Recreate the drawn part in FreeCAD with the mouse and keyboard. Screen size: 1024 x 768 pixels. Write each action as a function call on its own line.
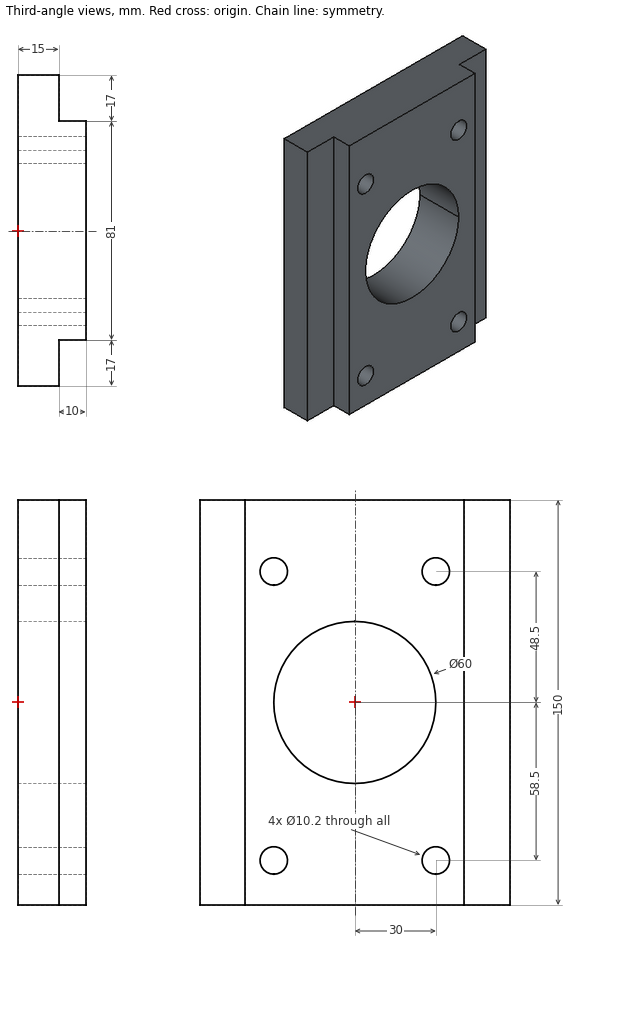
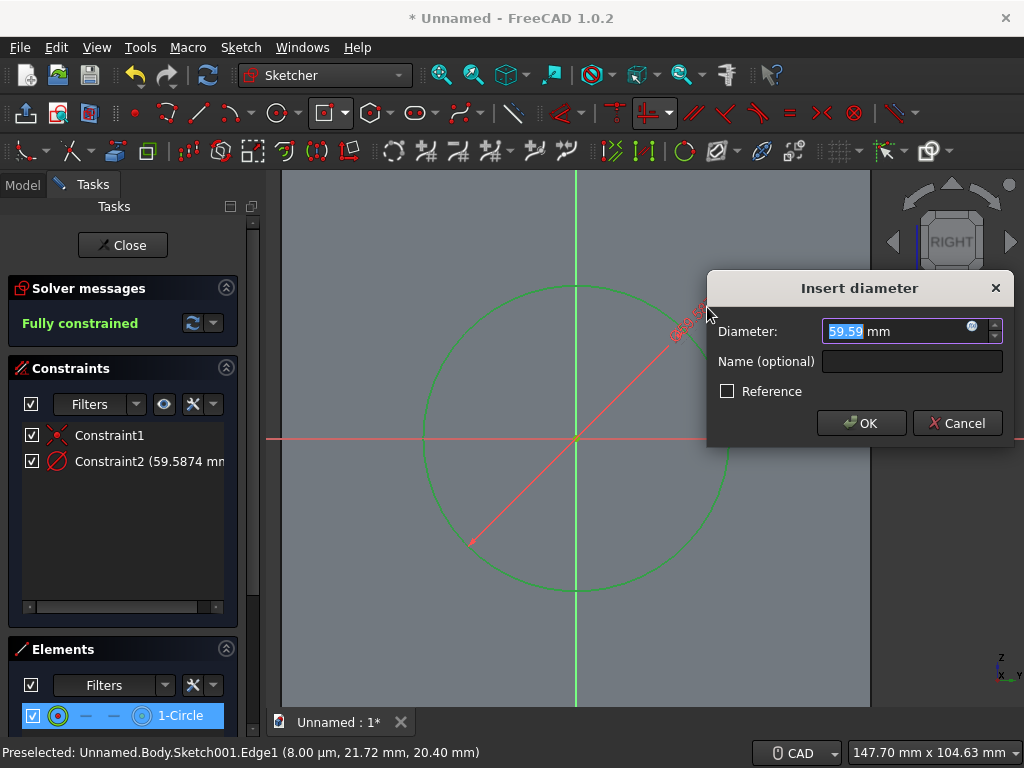
text(60)
key(Return)
key(Escape)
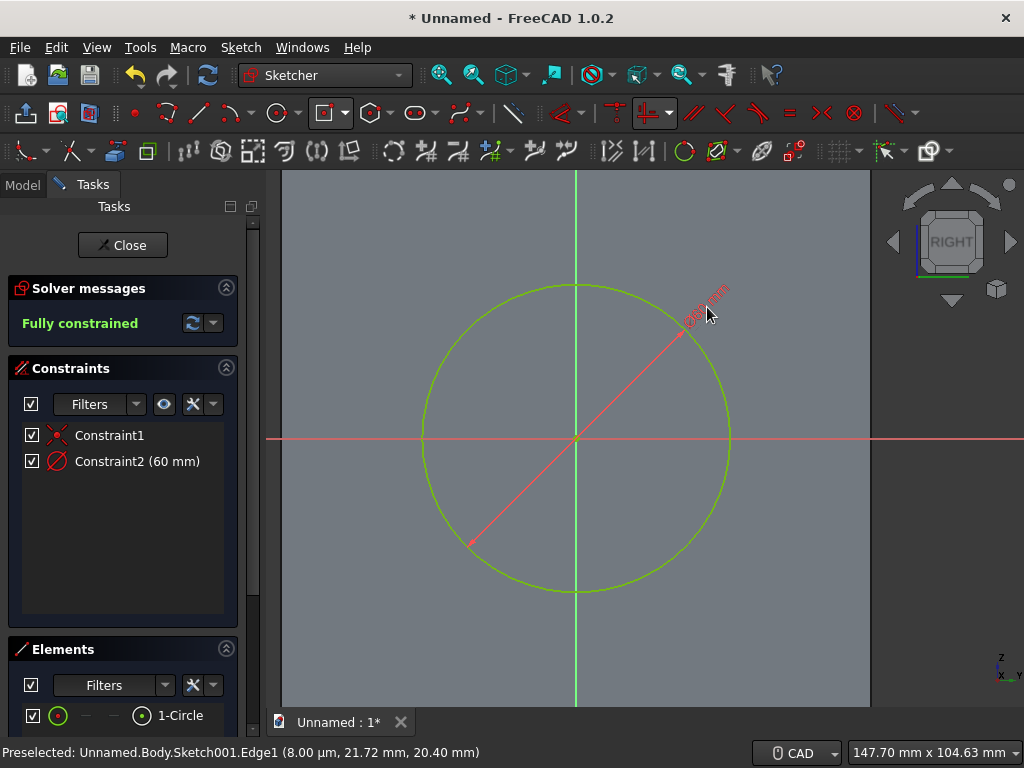
click(123, 245)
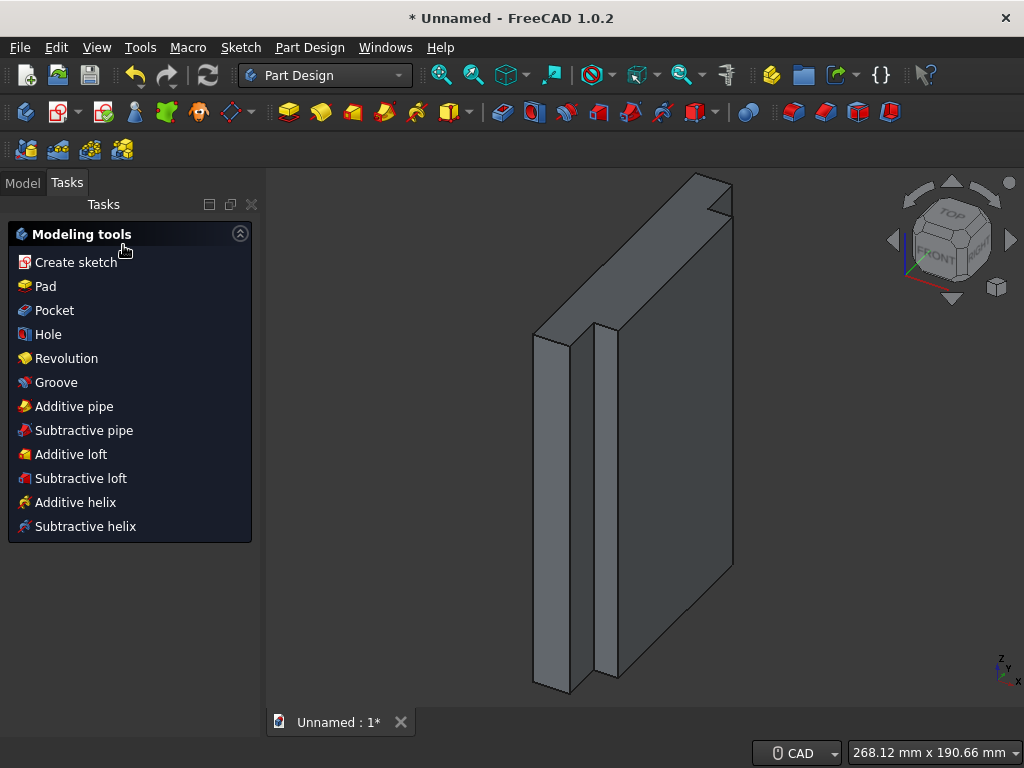
click(504, 112)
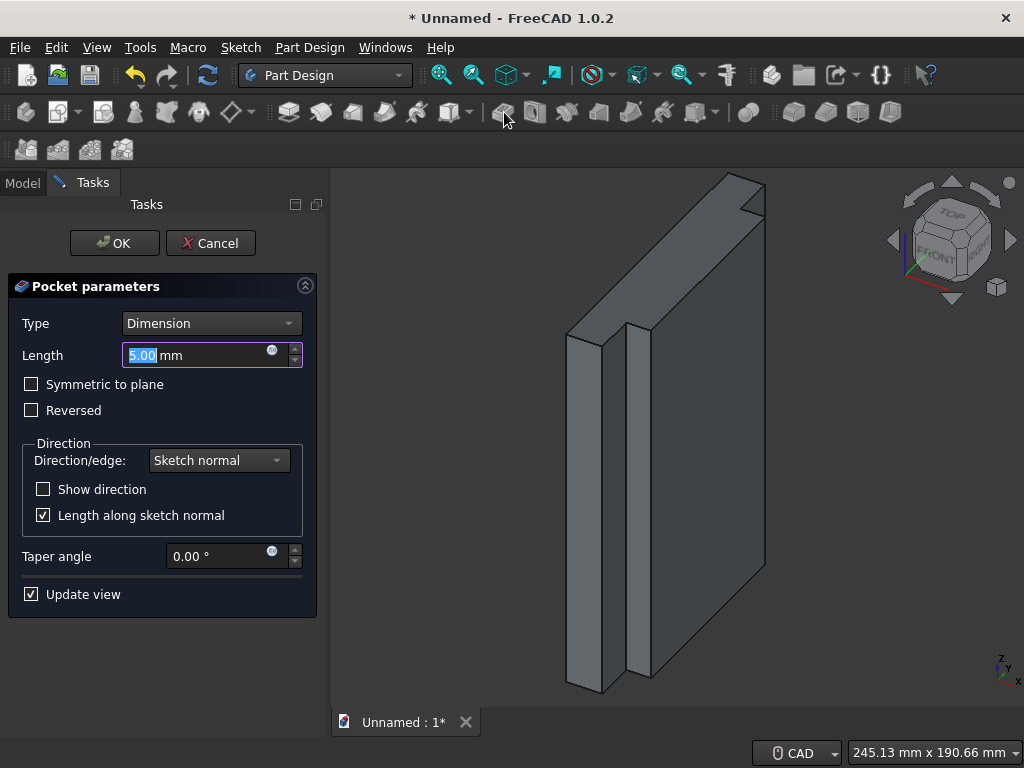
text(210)
key(Tab)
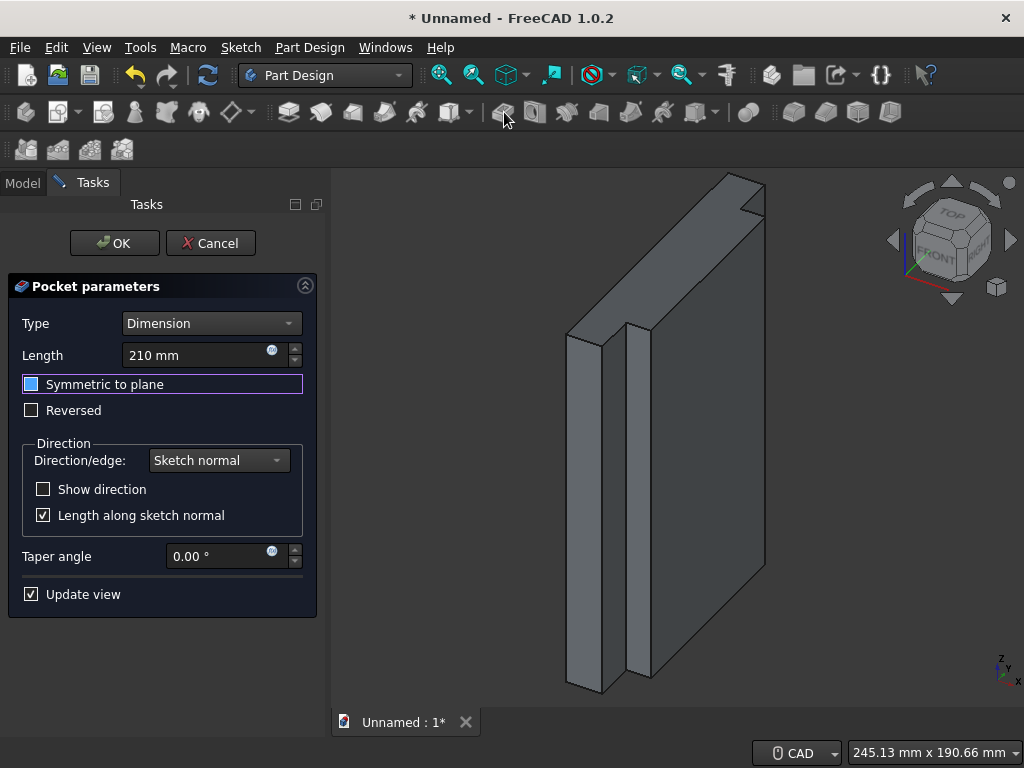
click(30, 410)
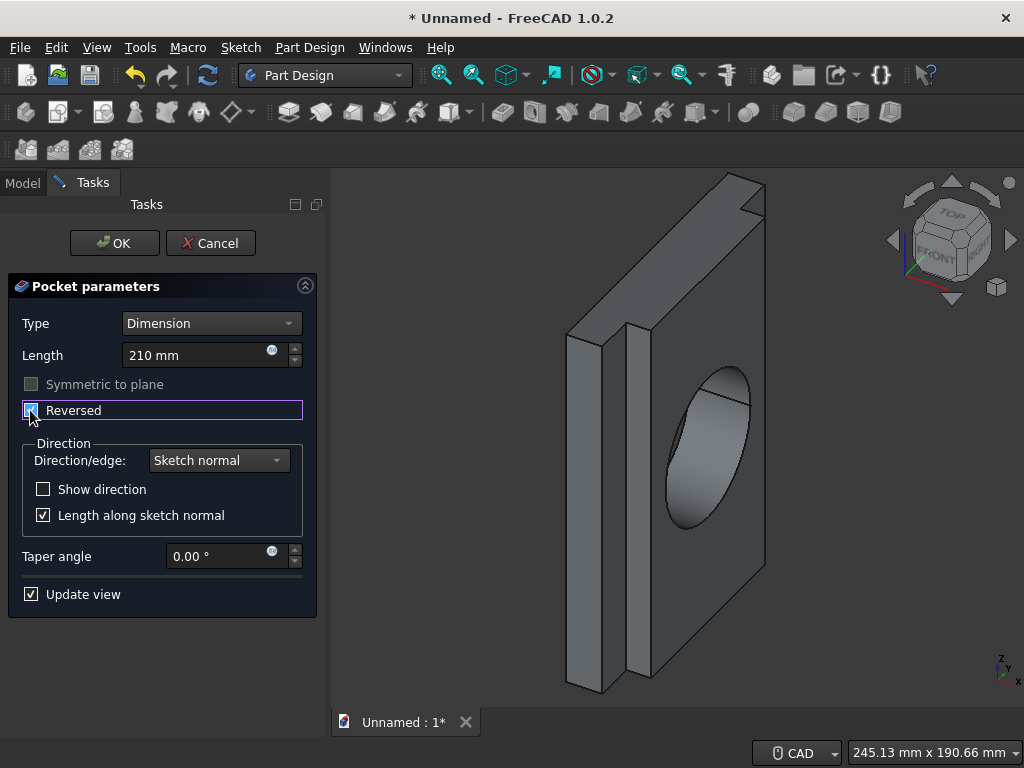
click(115, 243)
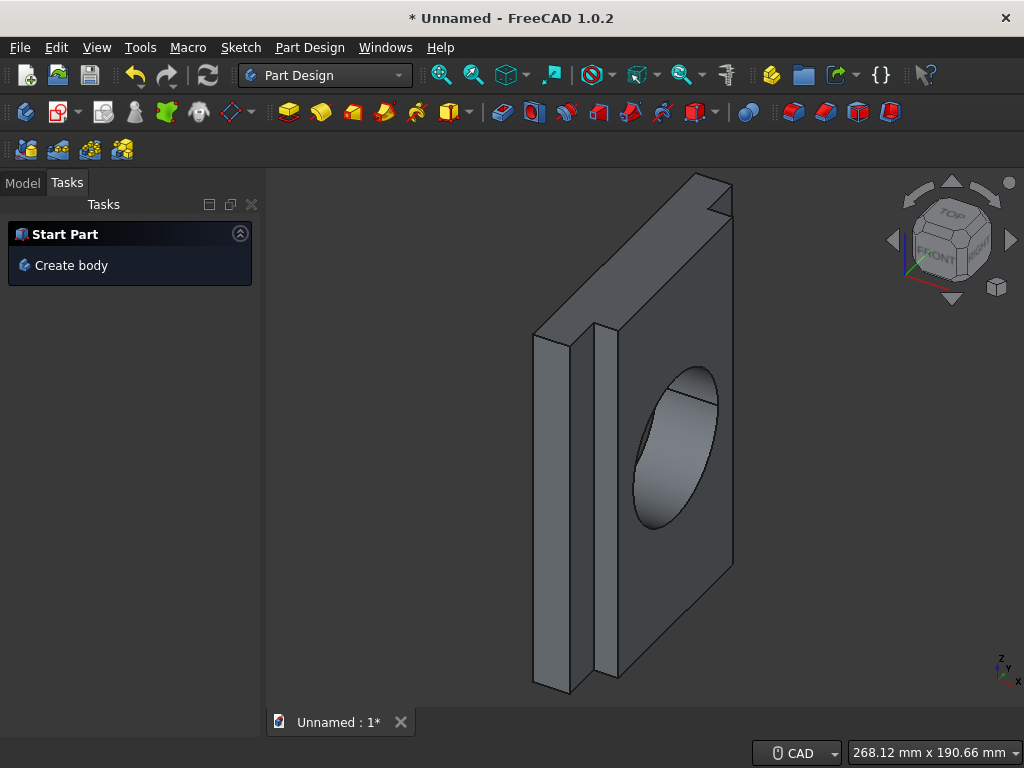
key(6)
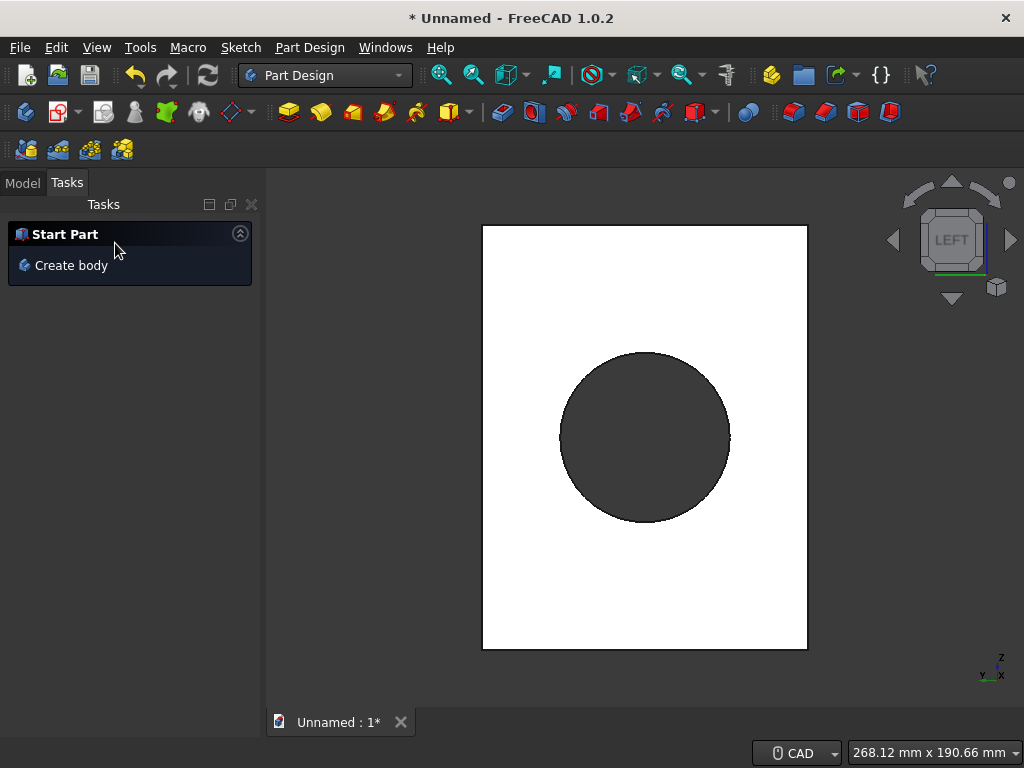
click(552, 315)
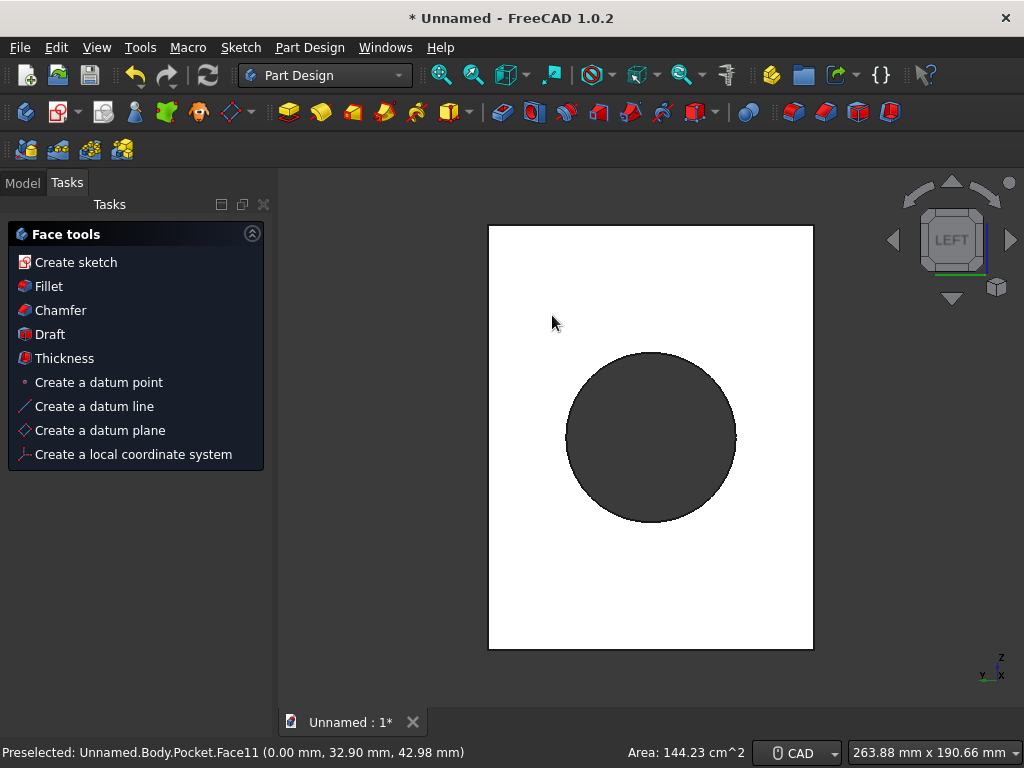
click(58, 112)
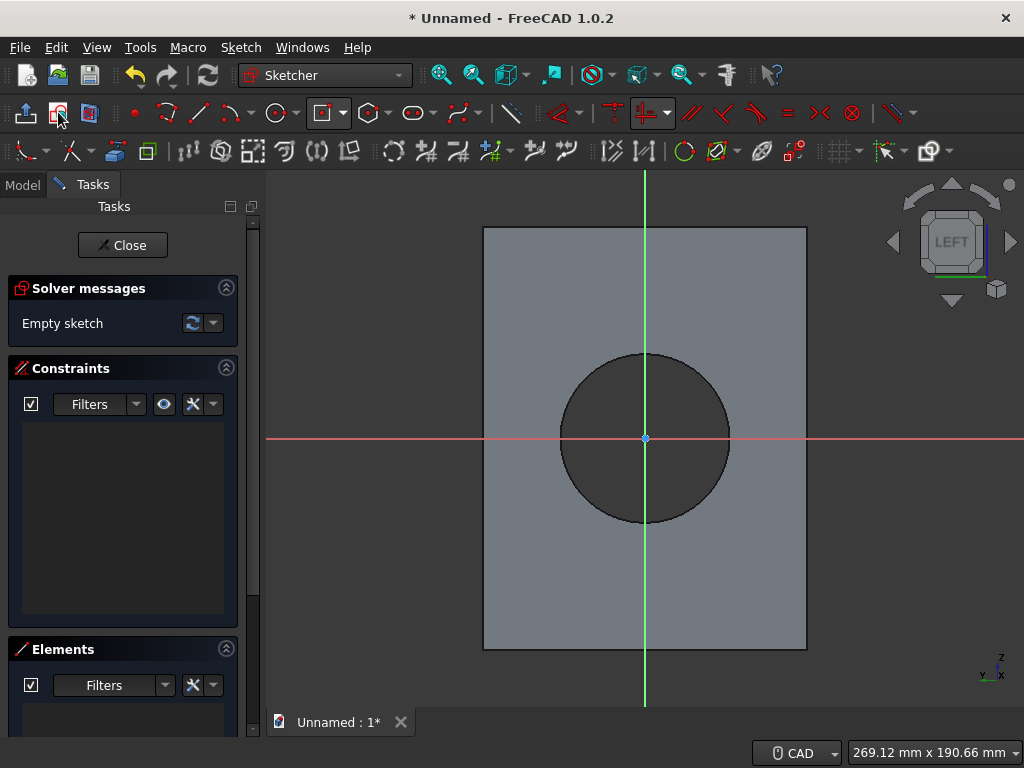
key(g)
key(c)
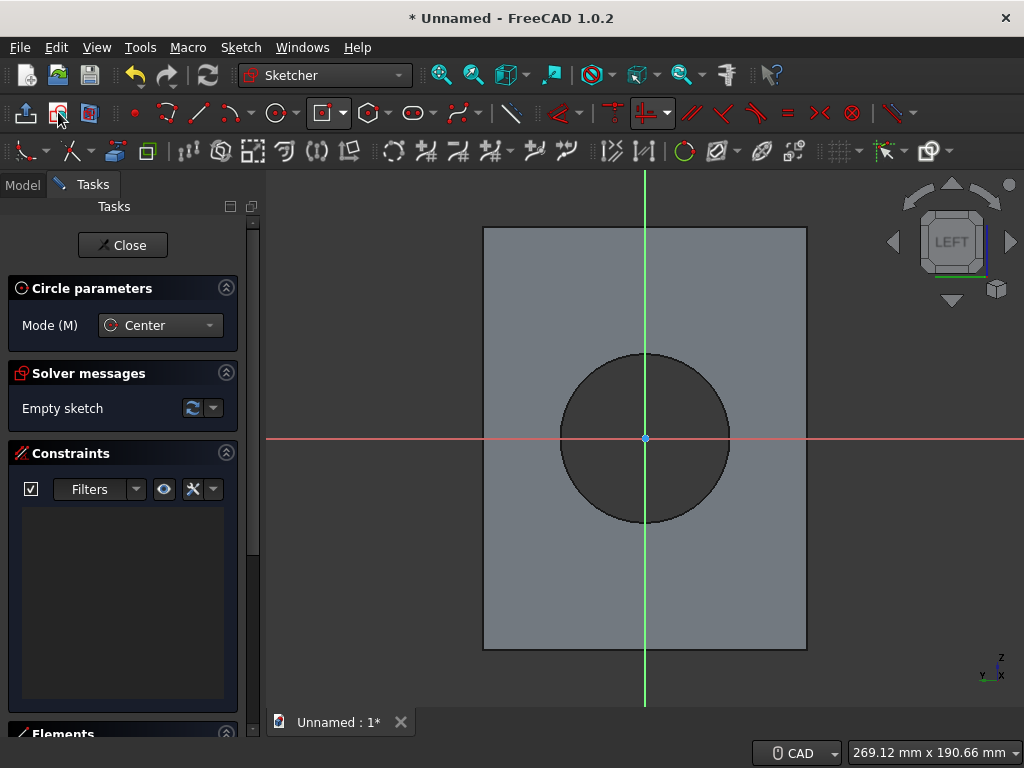
scroll(561, 603, up, 3)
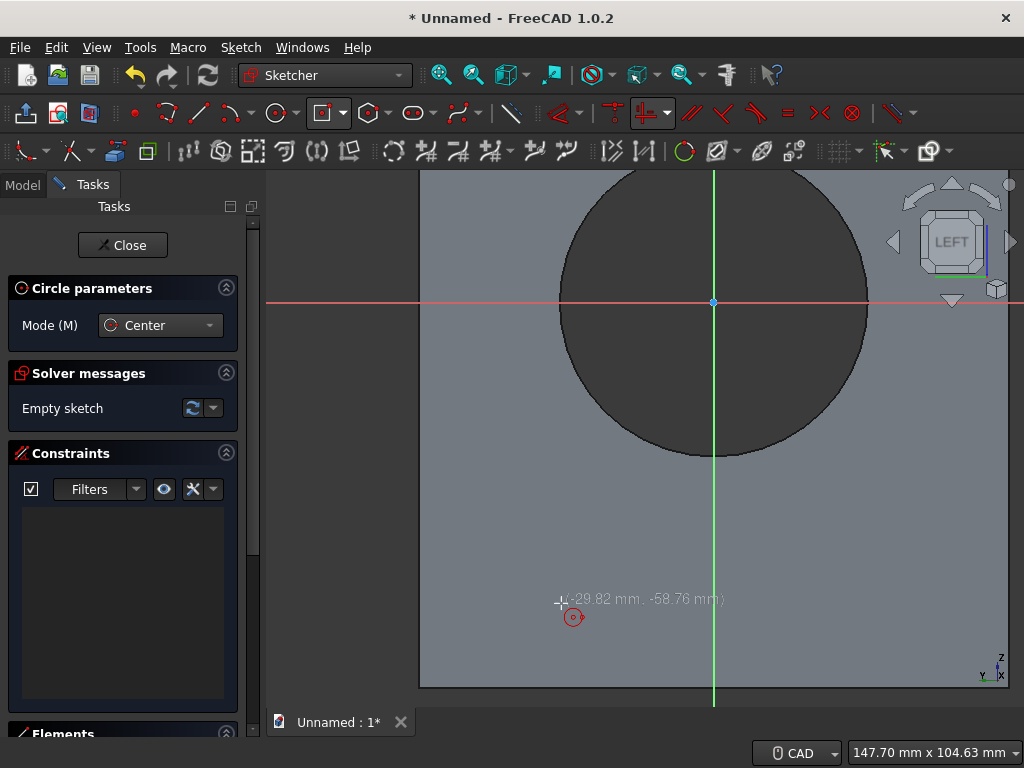
click(560, 603)
click(578, 584)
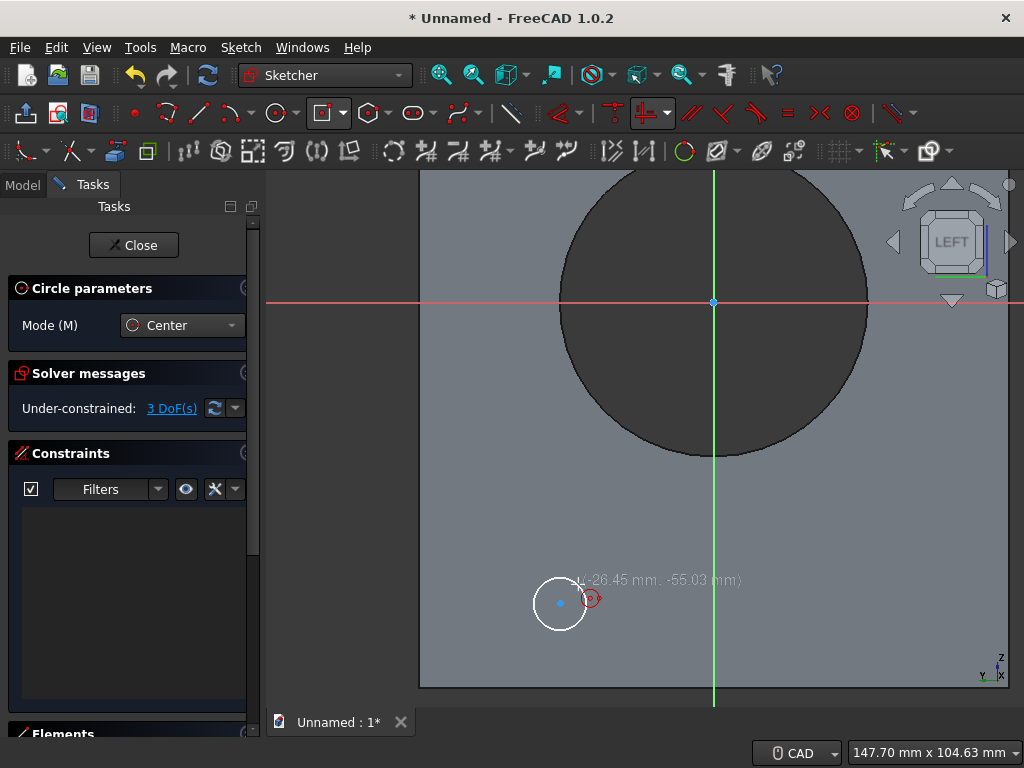
scroll(410, 573, down, 3)